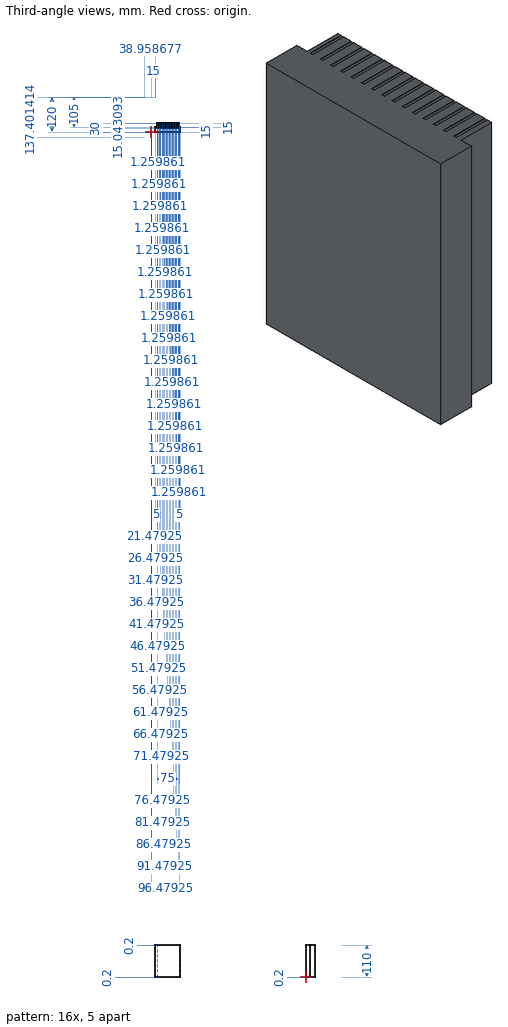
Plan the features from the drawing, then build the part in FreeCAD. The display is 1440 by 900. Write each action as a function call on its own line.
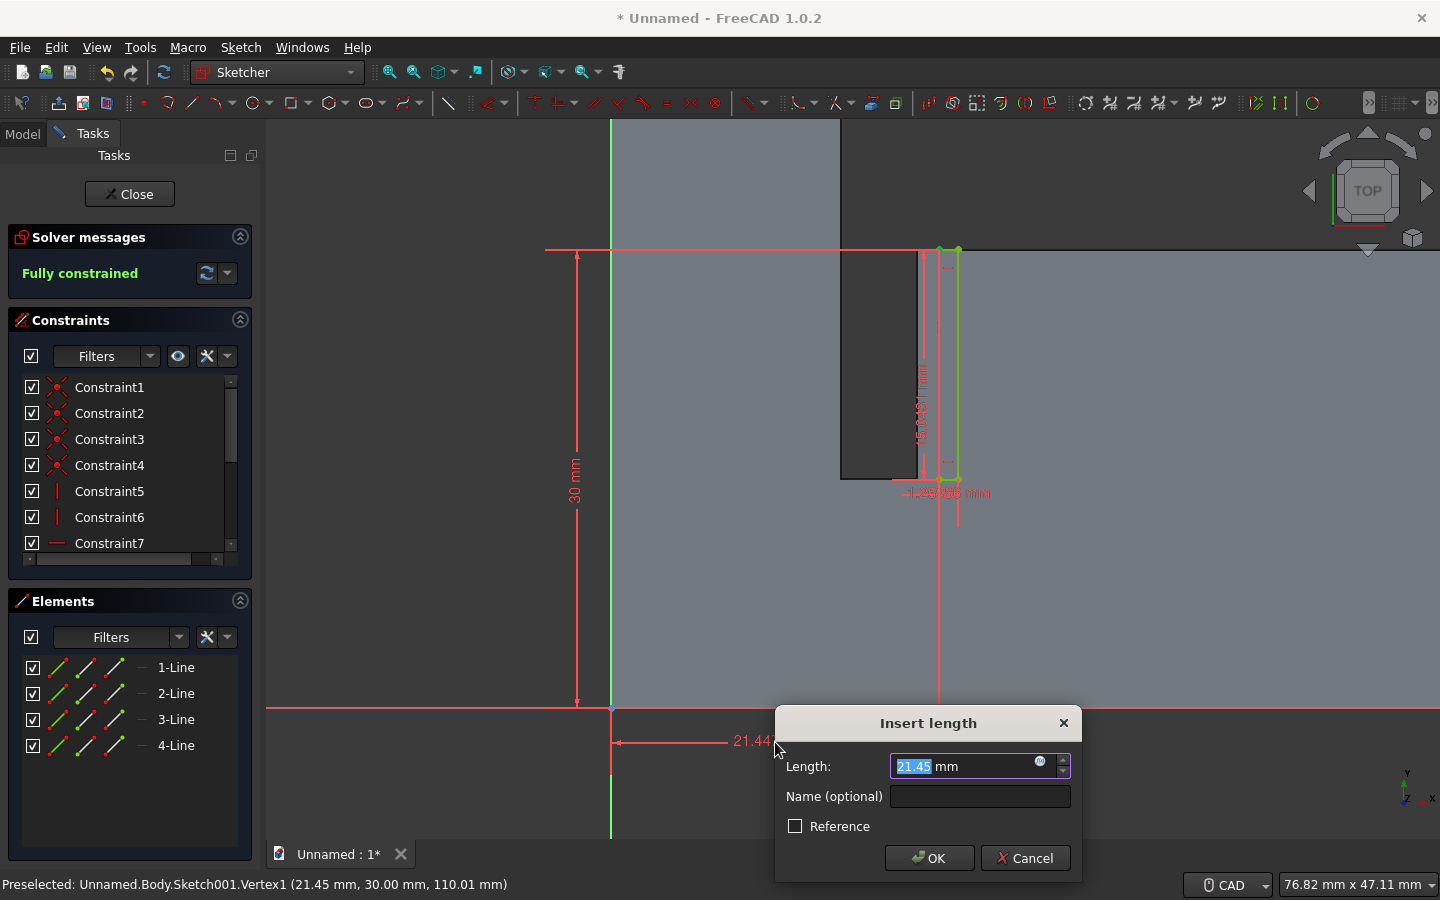
text(21.47925)
key(Return)
key(Escape)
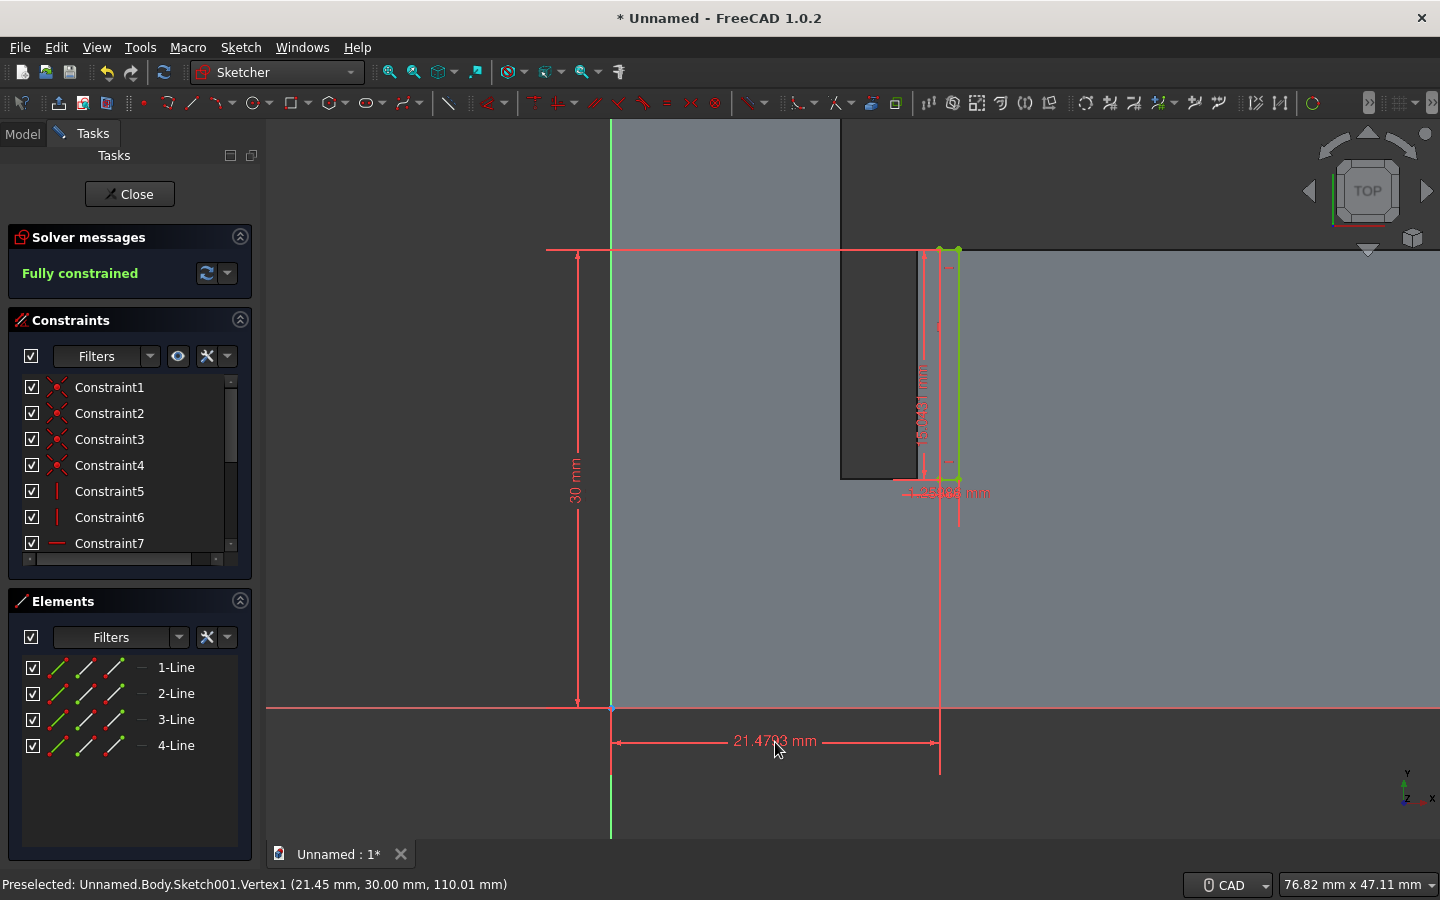
click(130, 194)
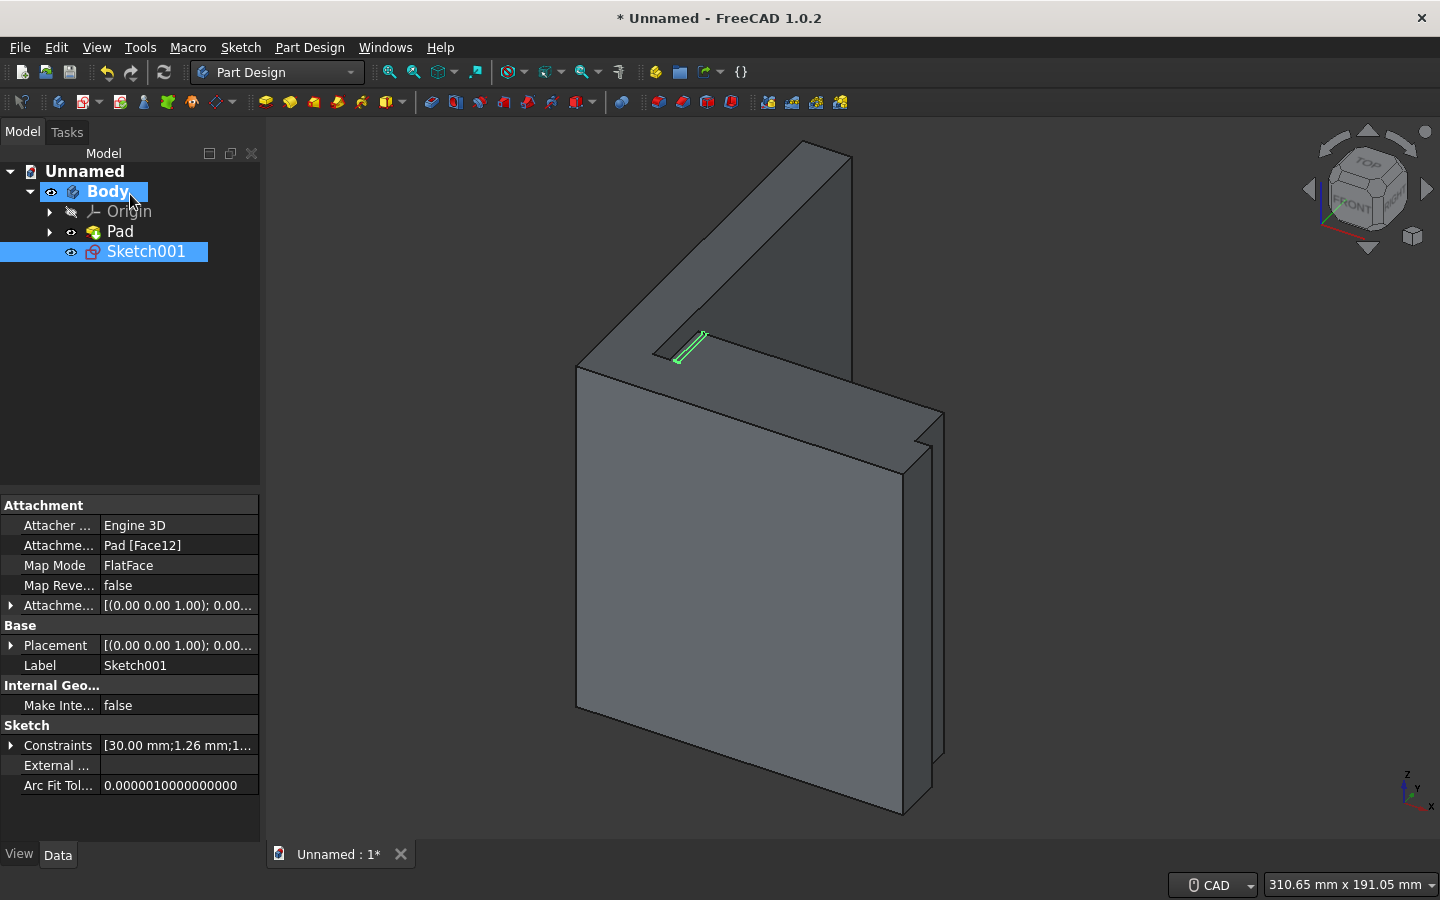
click(432, 102)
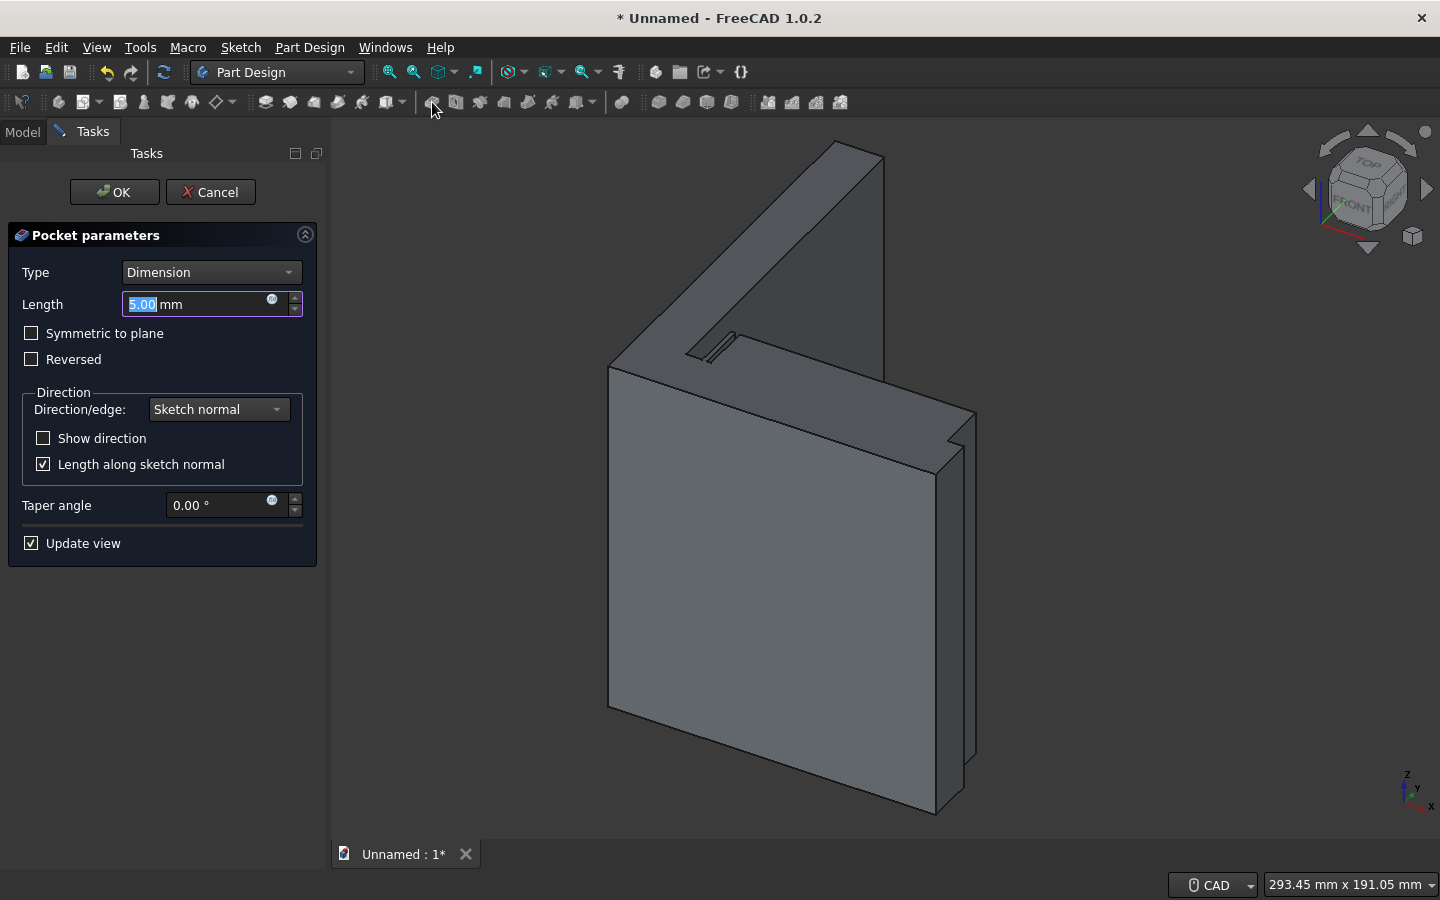
text(0.2)
key(Tab)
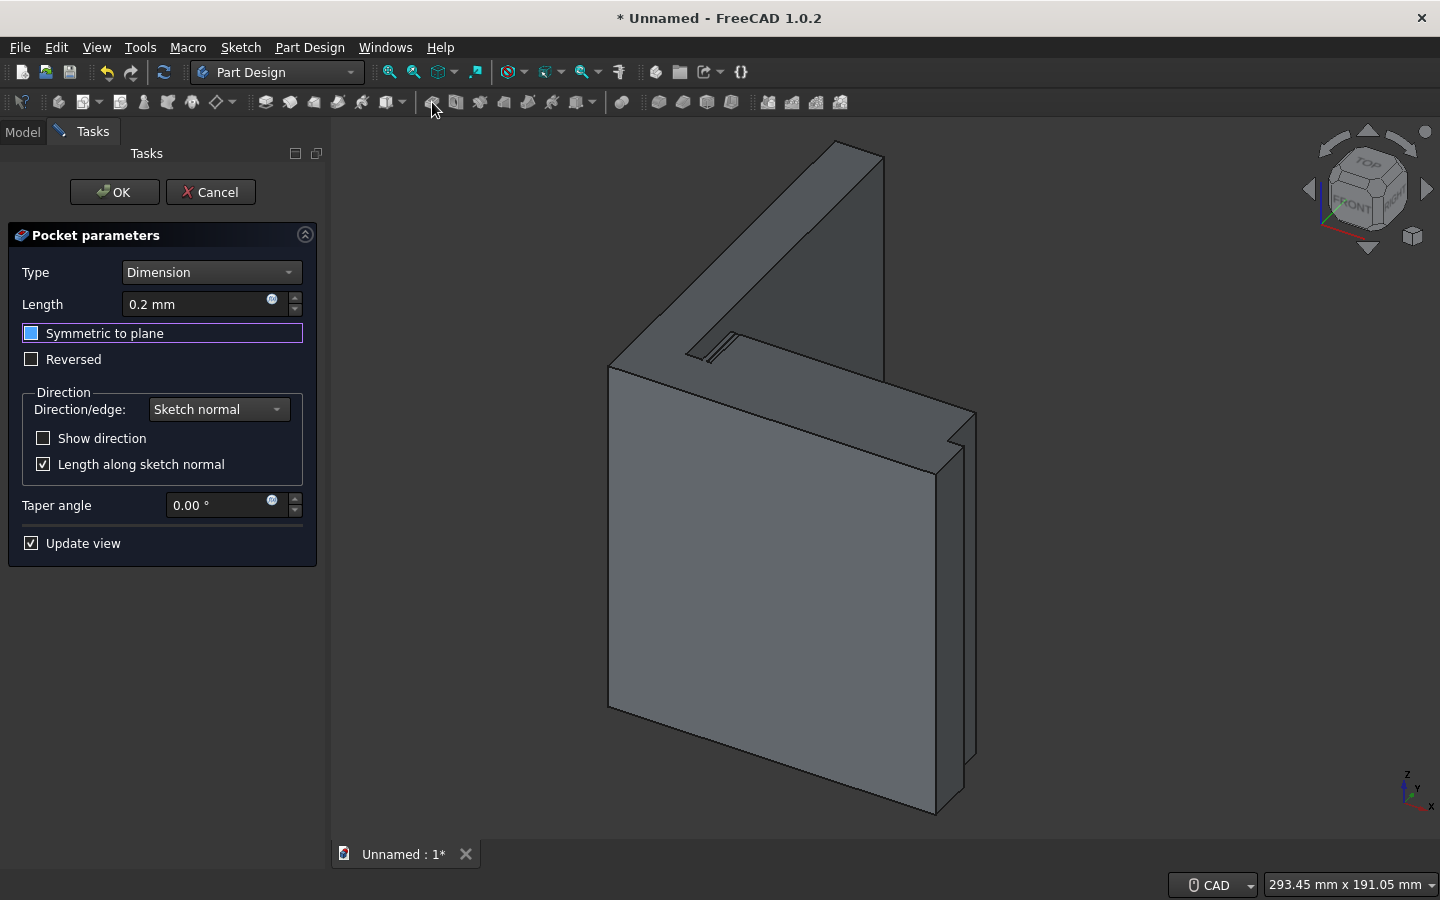
click(115, 192)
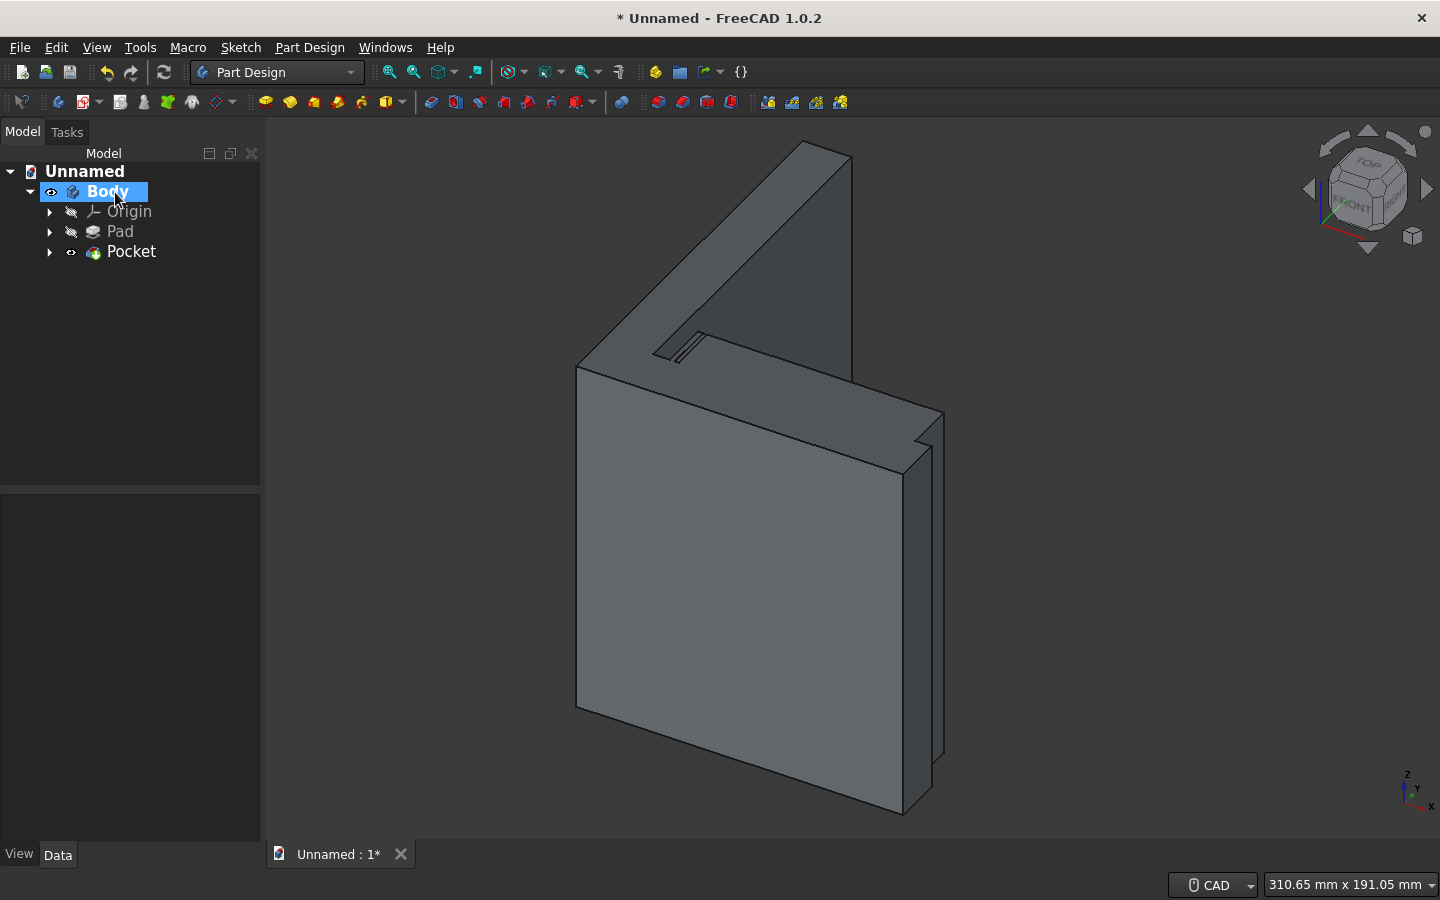
click(116, 252)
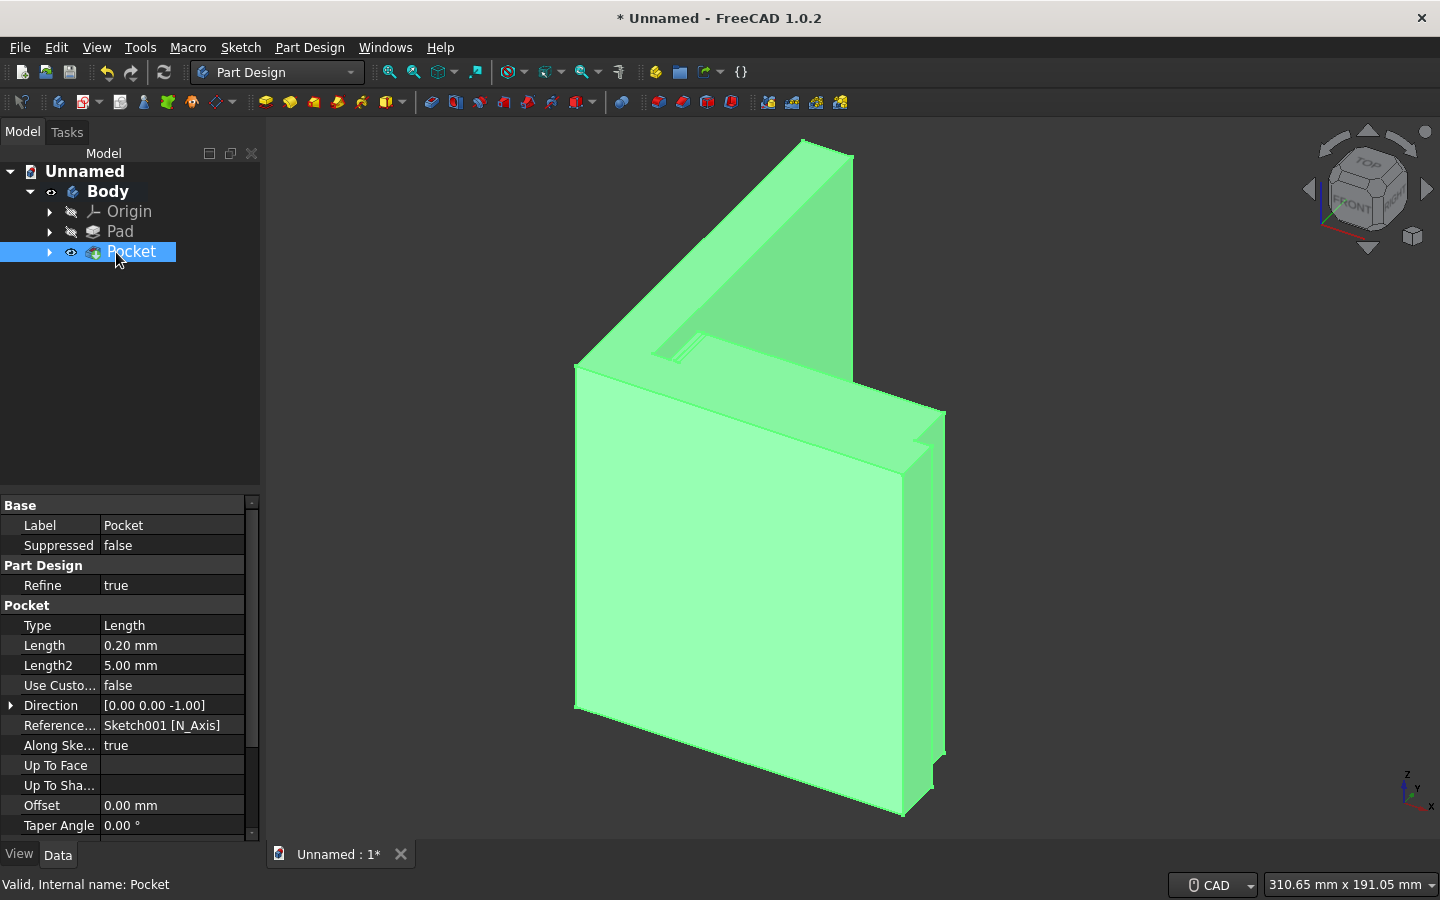
click(792, 102)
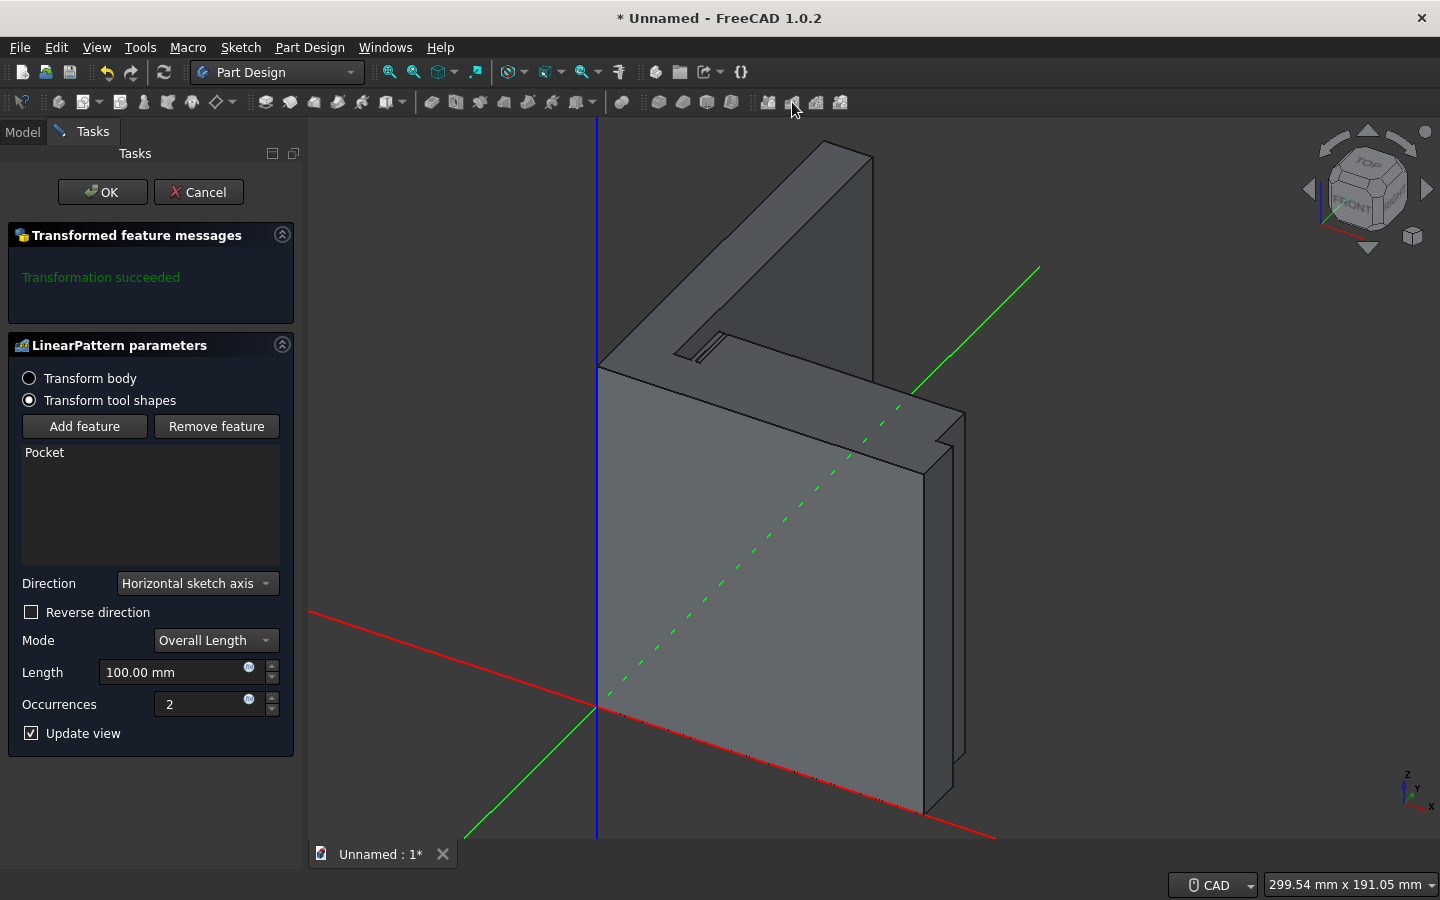
click(198, 584)